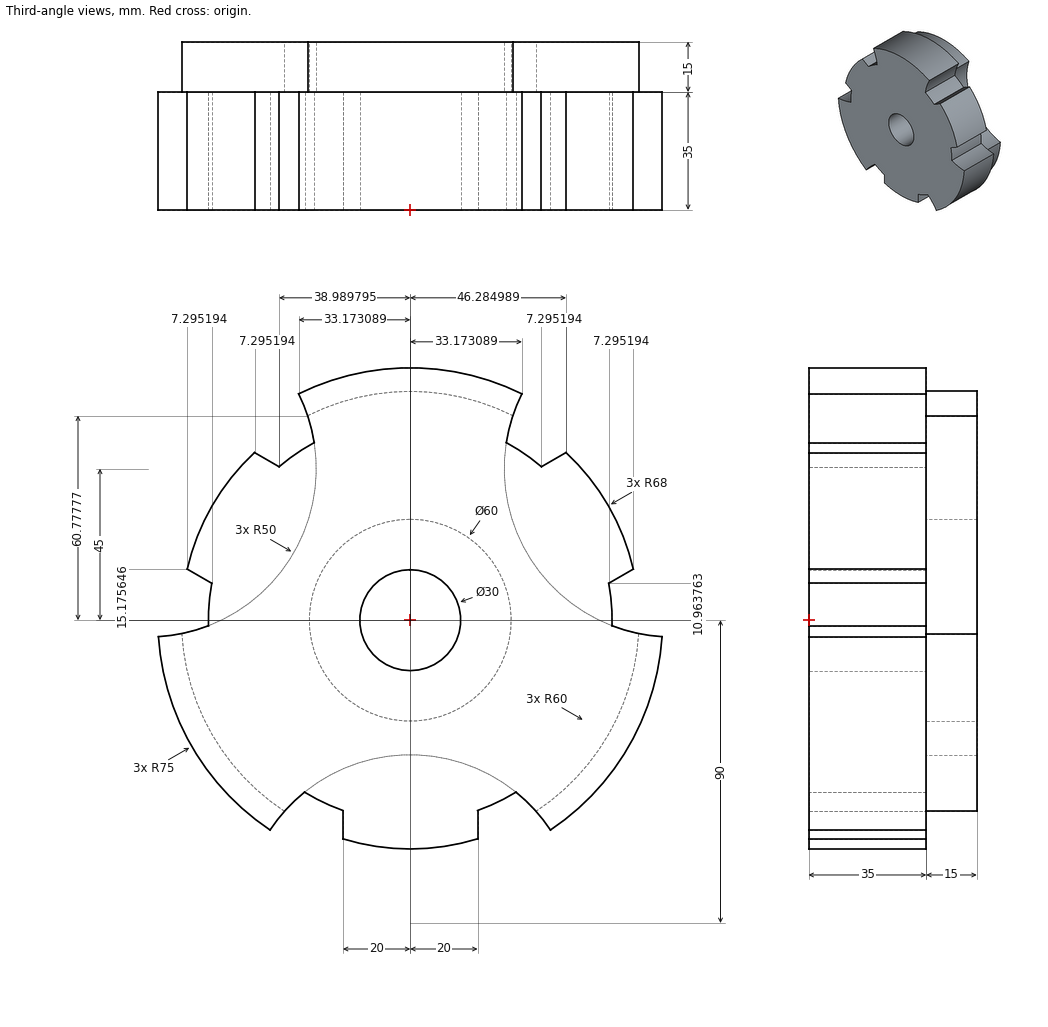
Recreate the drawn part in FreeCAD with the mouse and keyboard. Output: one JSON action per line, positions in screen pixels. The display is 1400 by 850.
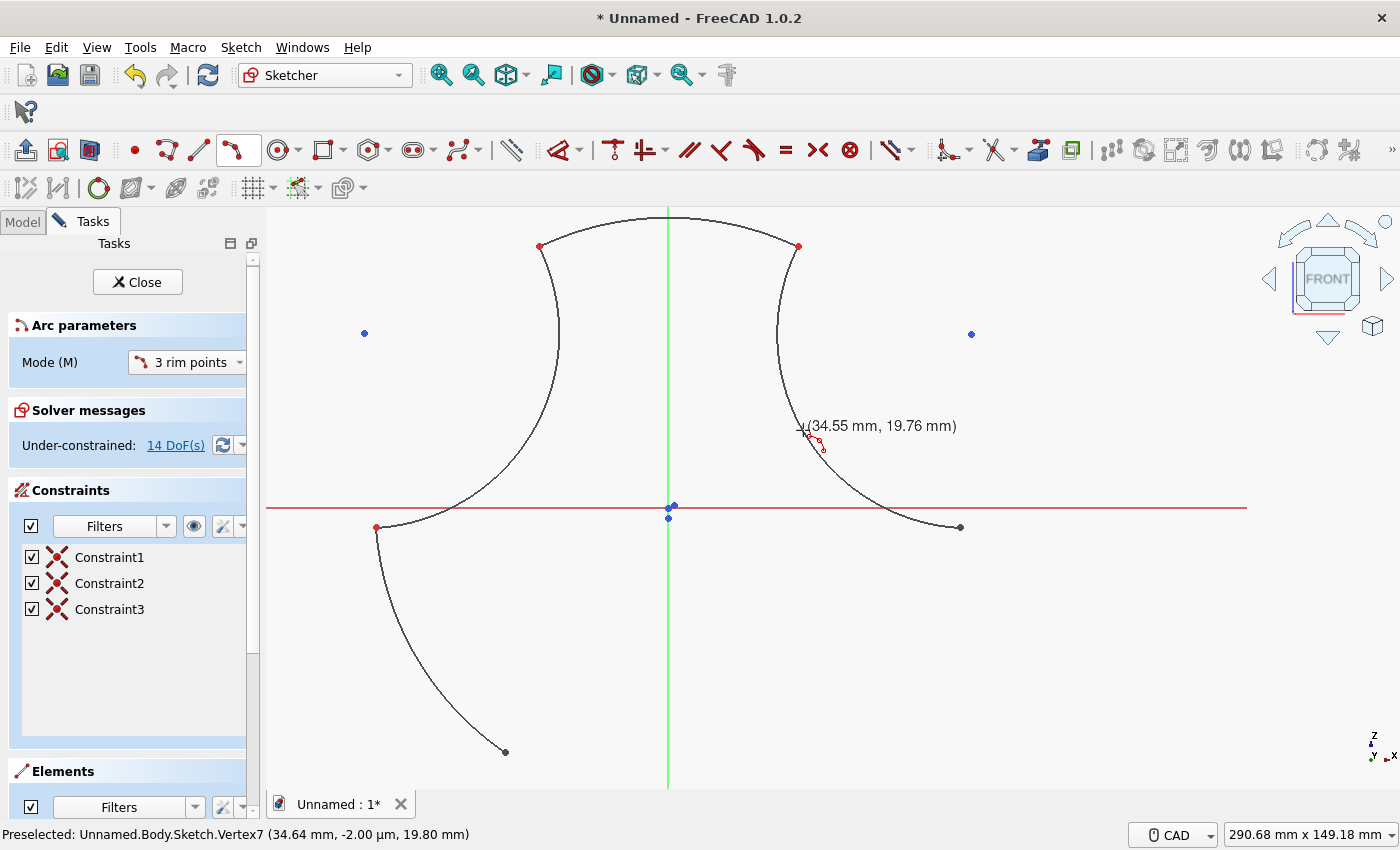
{"action": "left_click", "coordinate": [960, 528]}
{"action": "left_click", "coordinate": [831, 751]}
{"action": "left_click", "coordinate": [922, 654]}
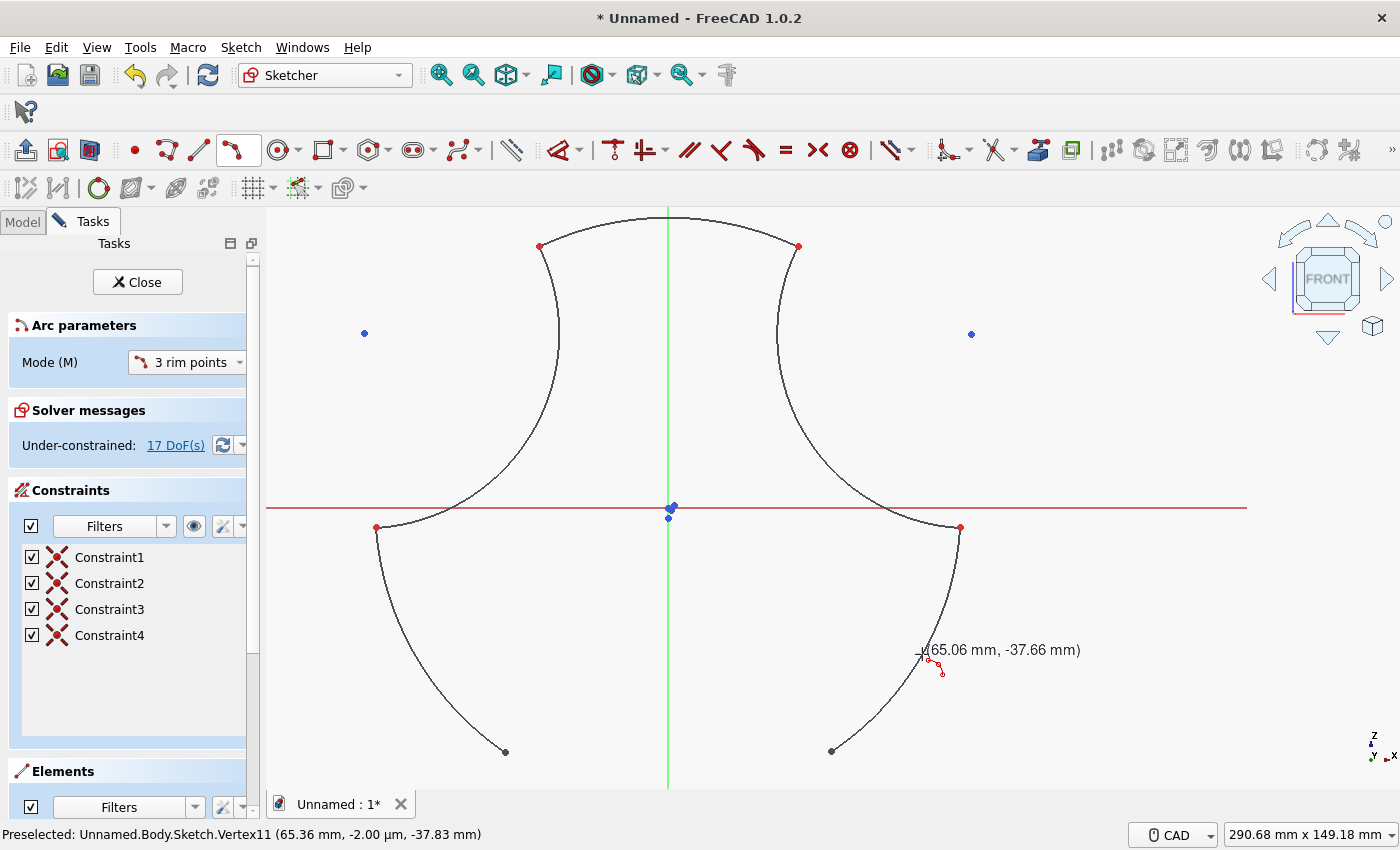
{"action": "left_click", "coordinate": [831, 752]}
{"action": "left_click", "coordinate": [506, 753]}
{"action": "left_click", "coordinate": [706, 668]}
{"action": "key", "text": "Escape"}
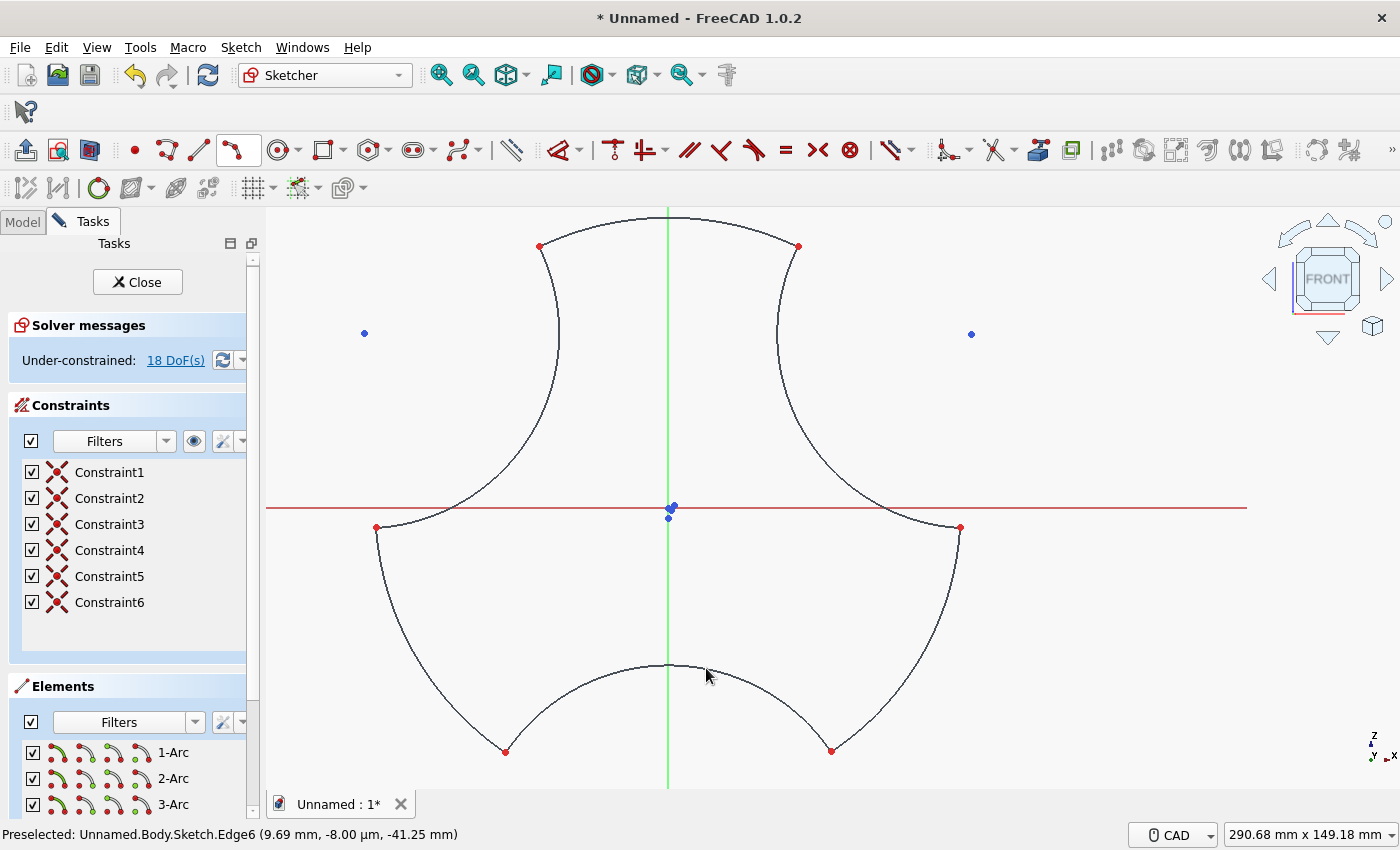
{"action": "left_click", "coordinate": [393, 607]}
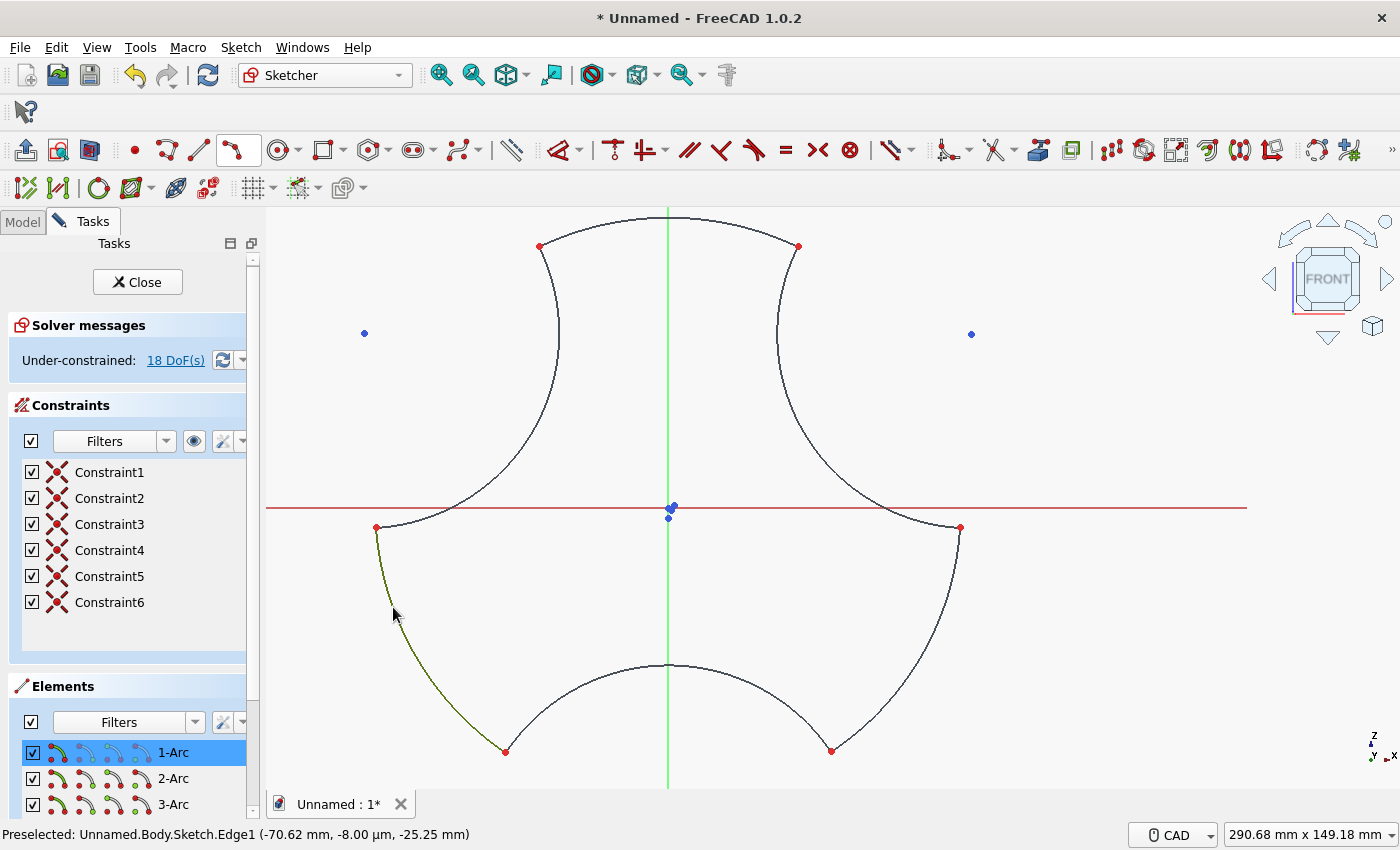
{"action": "scroll", "coordinate": [960, 528], "scroll_direction": "down", "scroll_amount": 2}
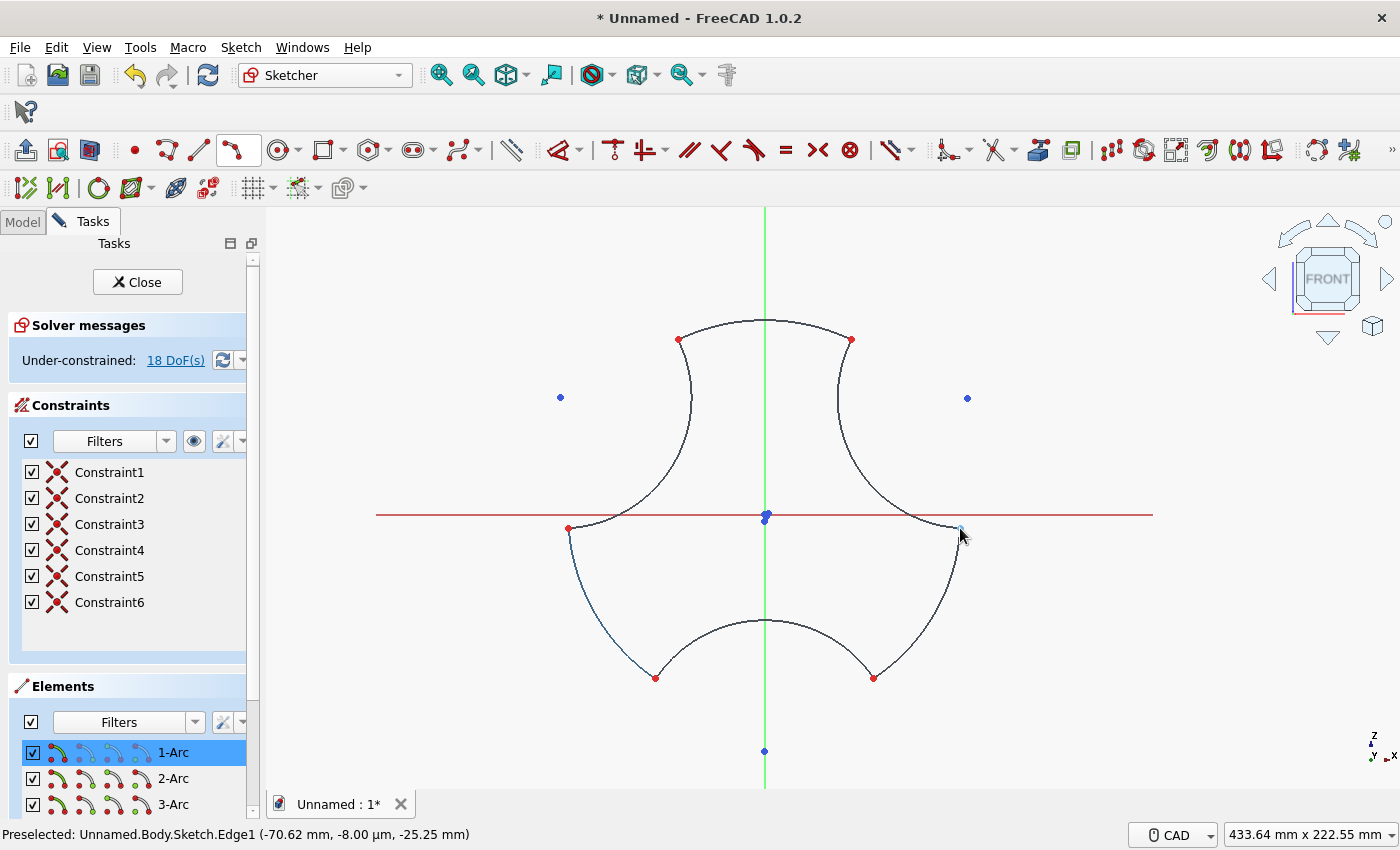
{"action": "left_click", "coordinate": [801, 323]}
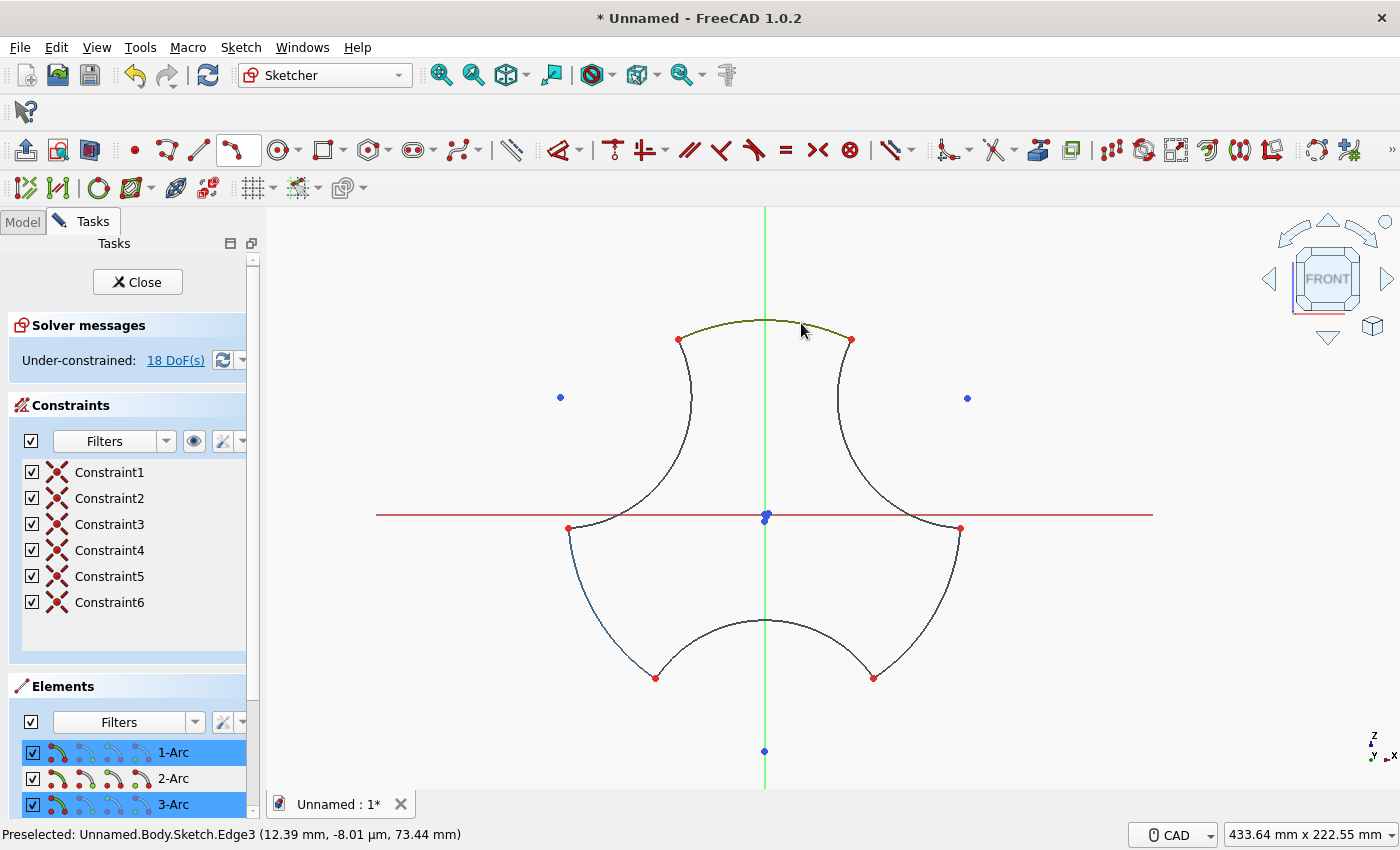
{"action": "left_click", "coordinate": [614, 150]}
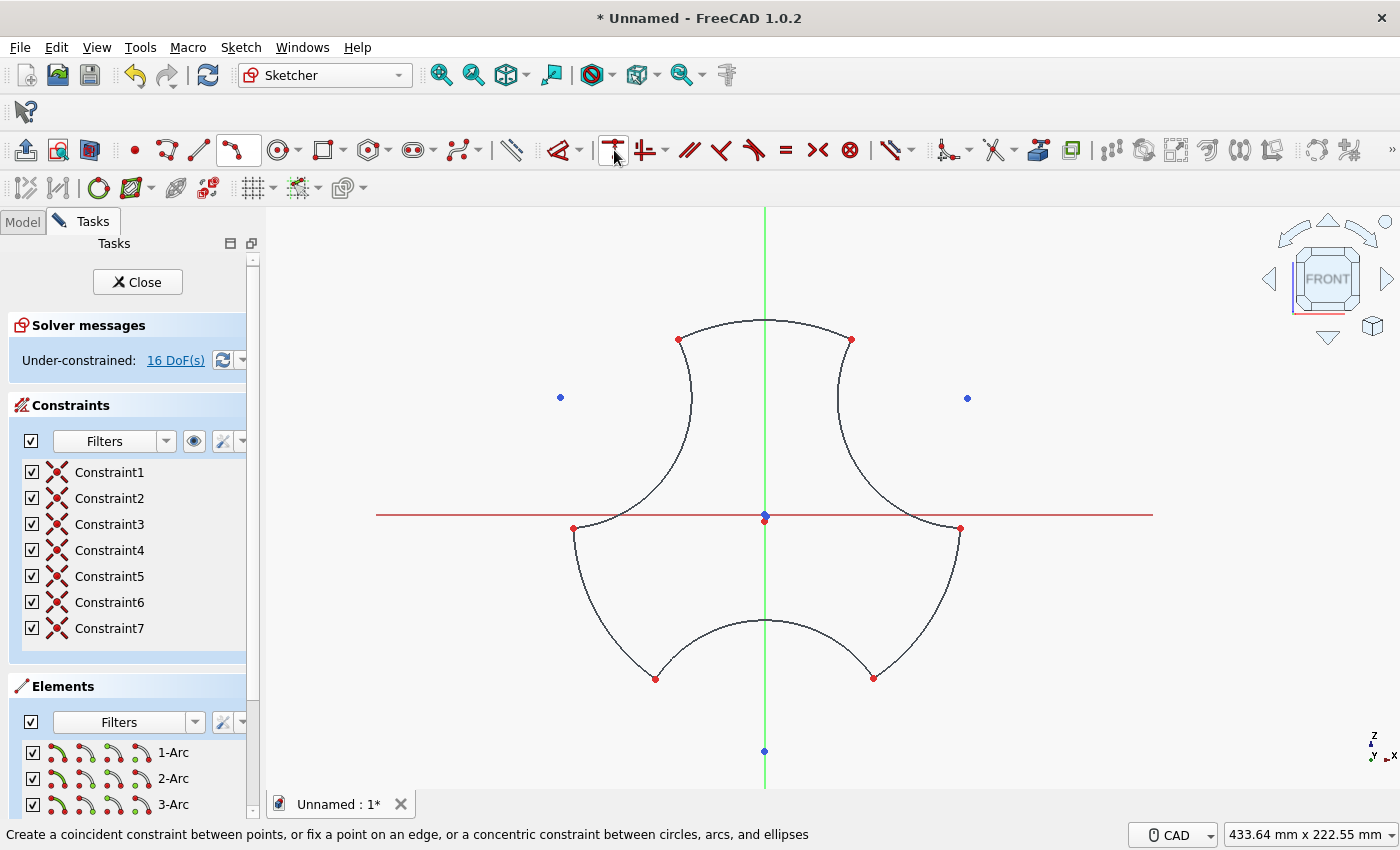
{"action": "left_click", "coordinate": [583, 581]}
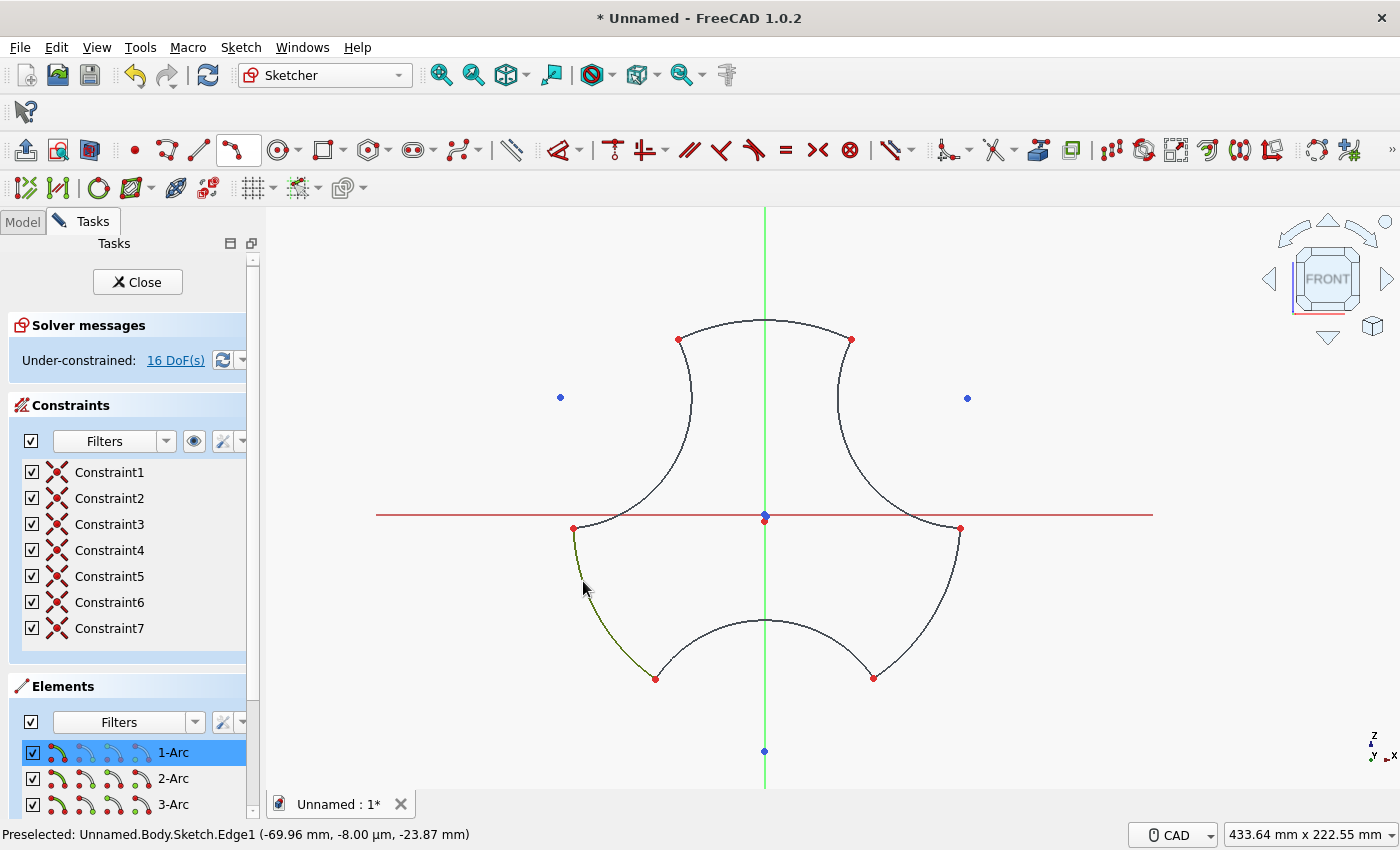
{"action": "left_click", "coordinate": [914, 643]}